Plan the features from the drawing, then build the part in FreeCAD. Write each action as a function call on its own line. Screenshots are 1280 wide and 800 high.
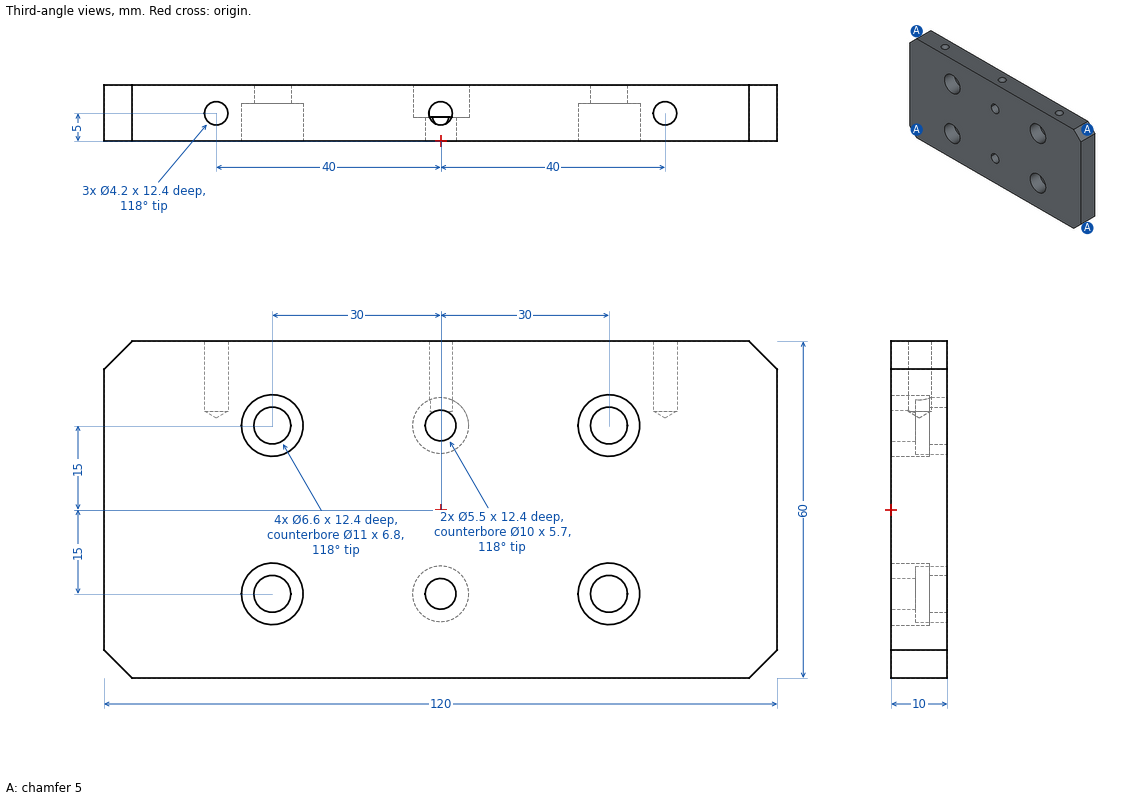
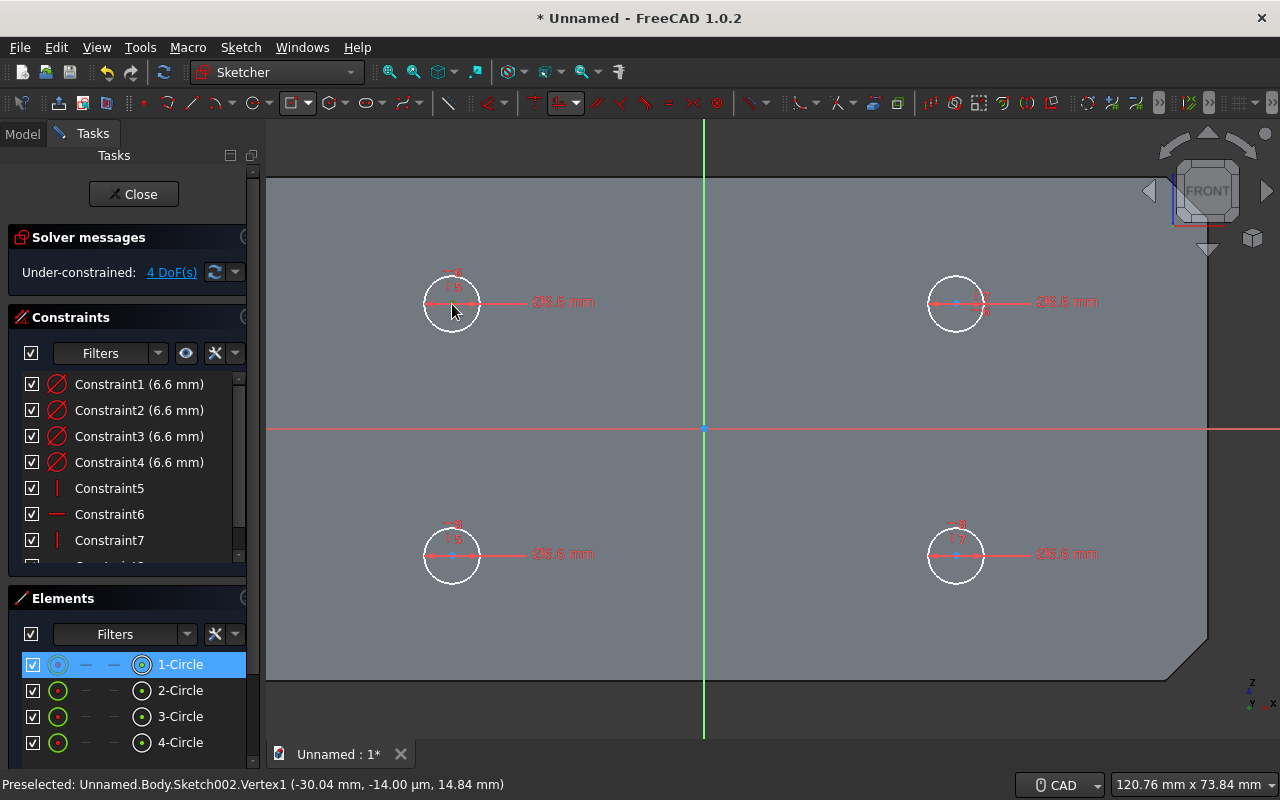
key(l)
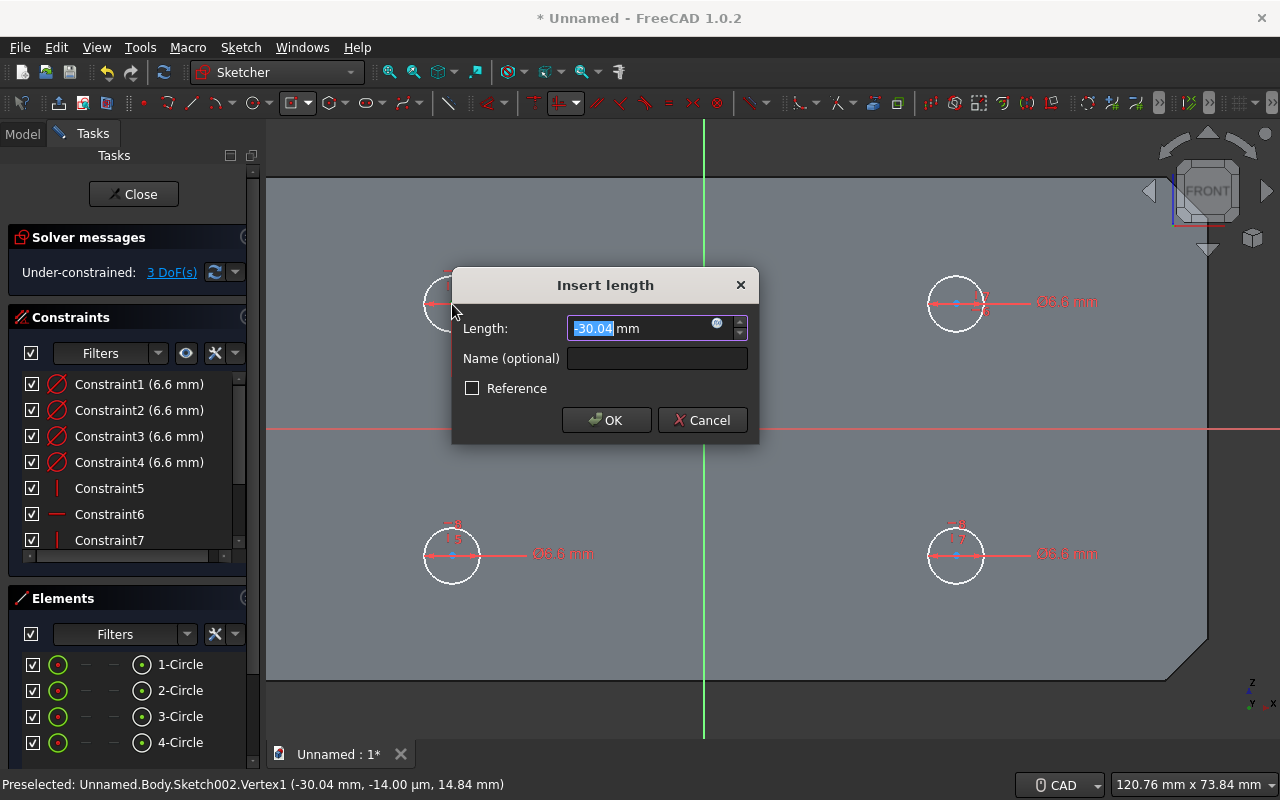
text(-30)
key(Return)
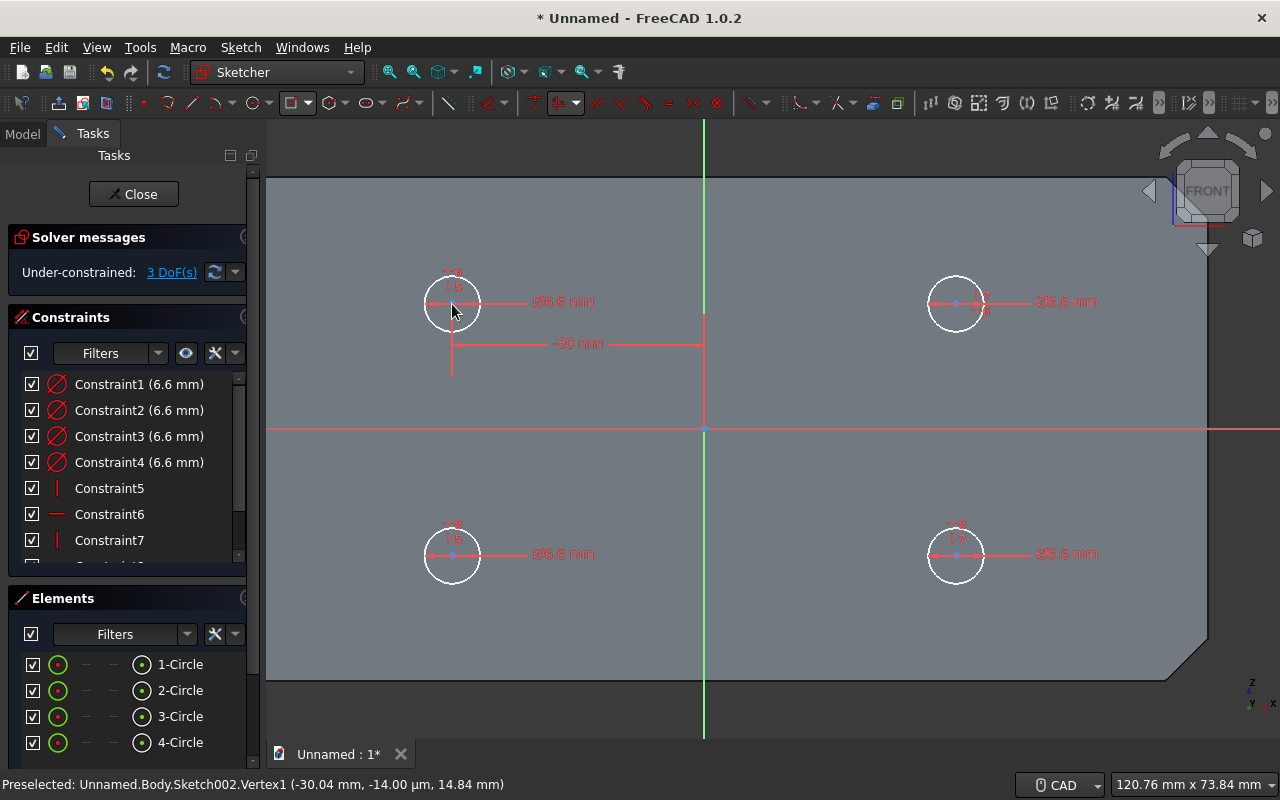
click(452, 304)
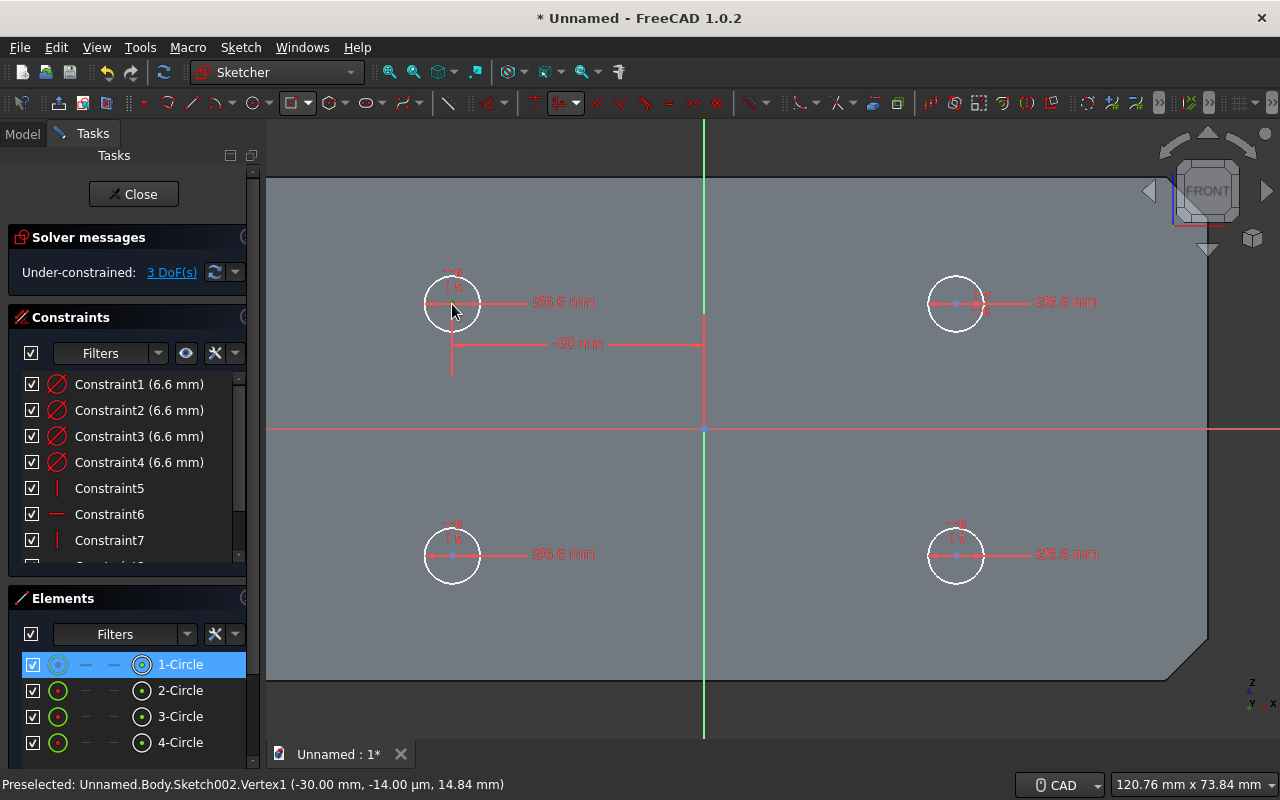
key(i)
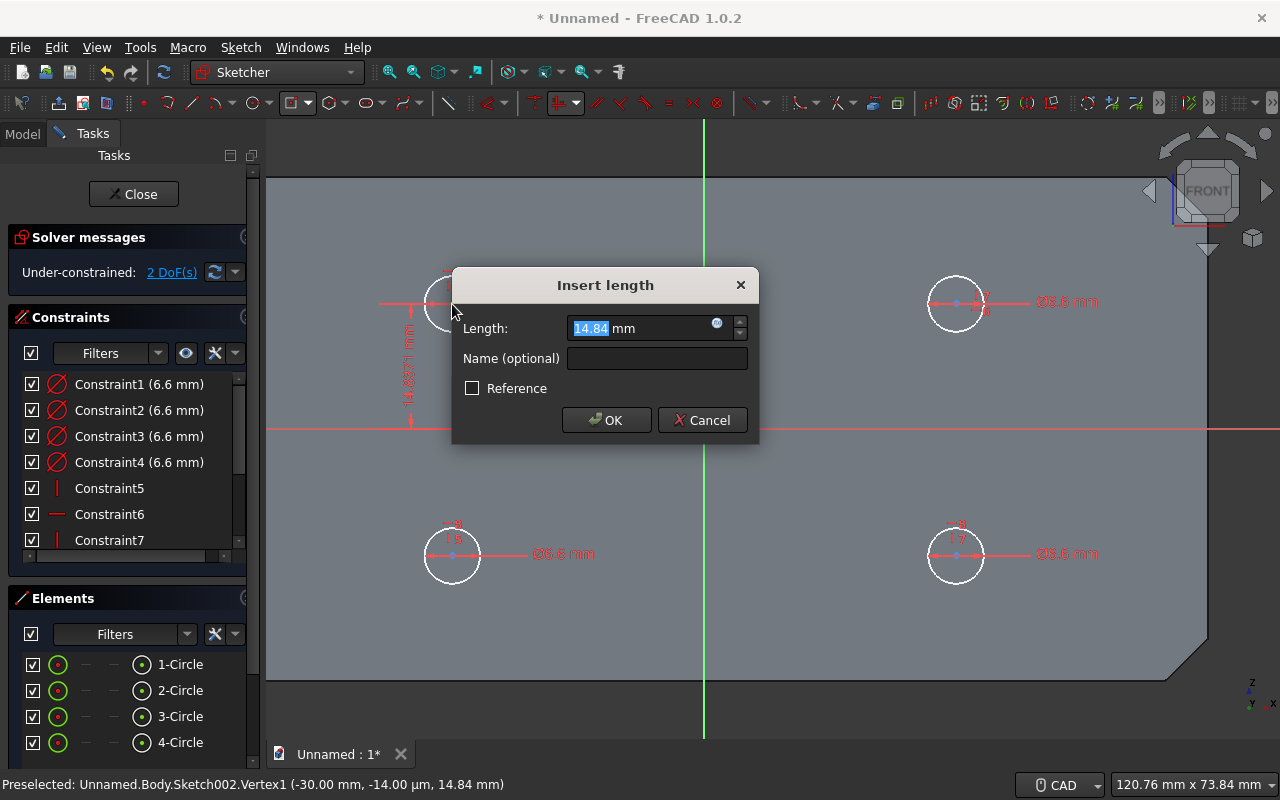
text(15)
key(Return)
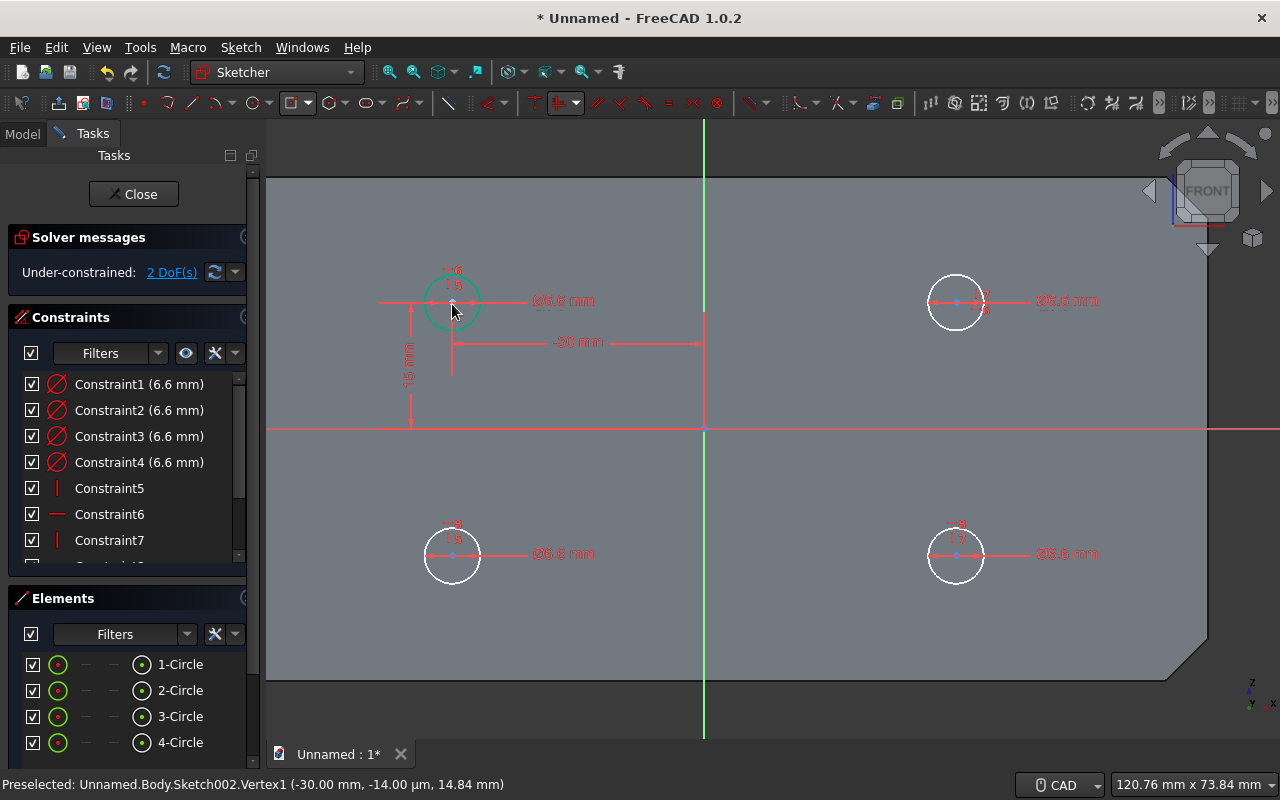
click(452, 556)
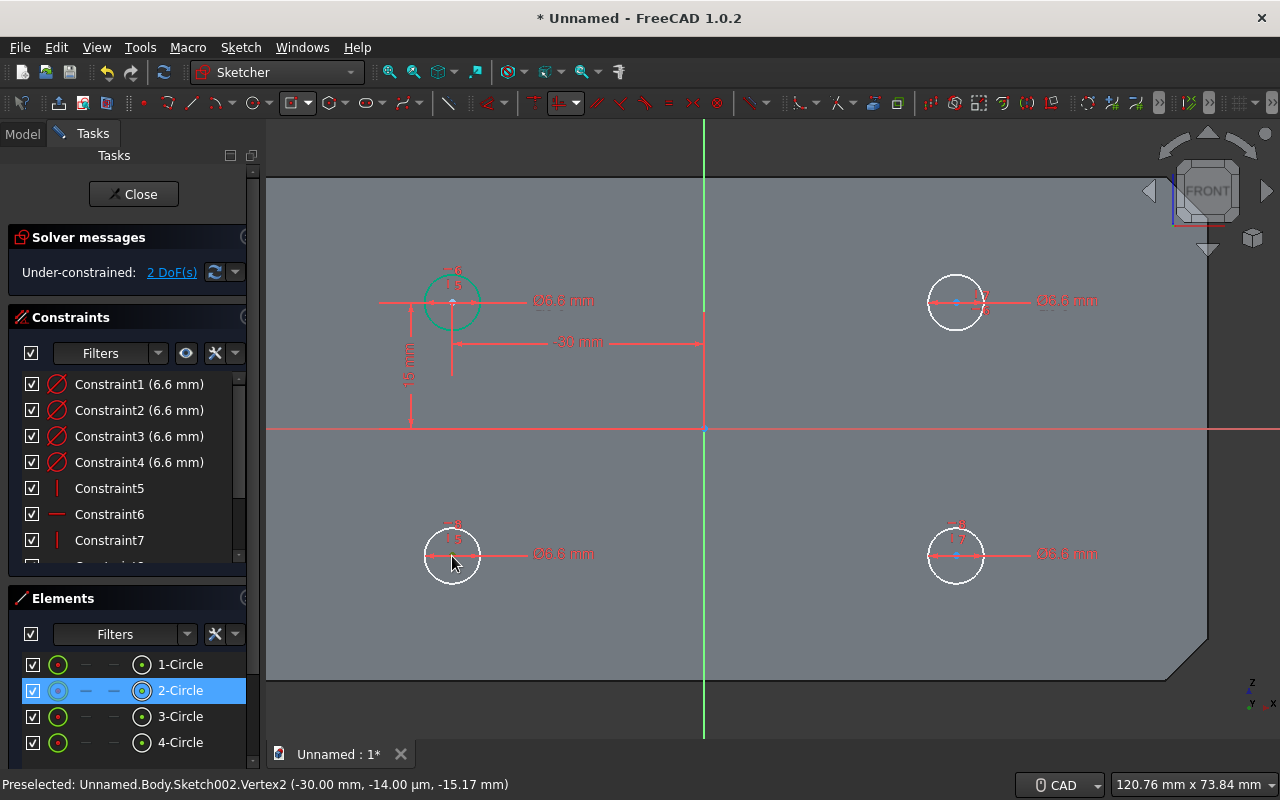
click(506, 104)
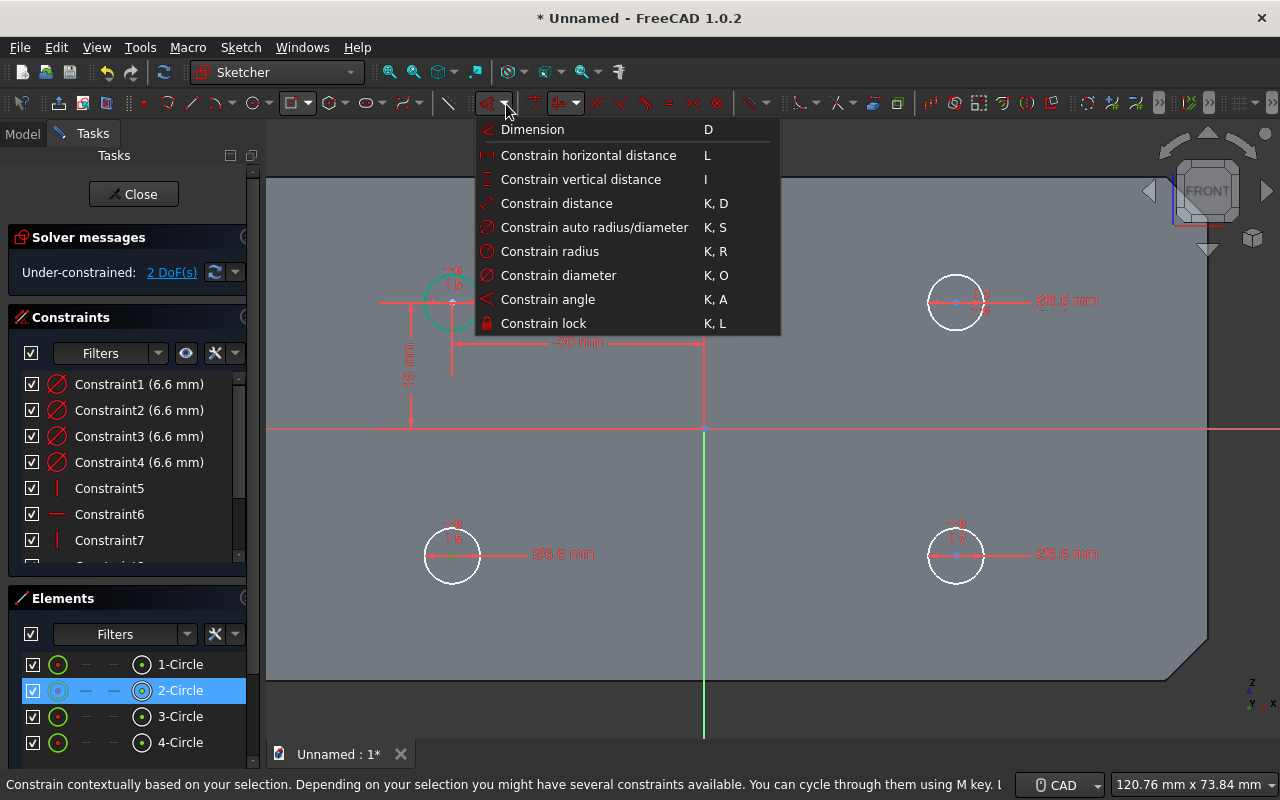
click(628, 179)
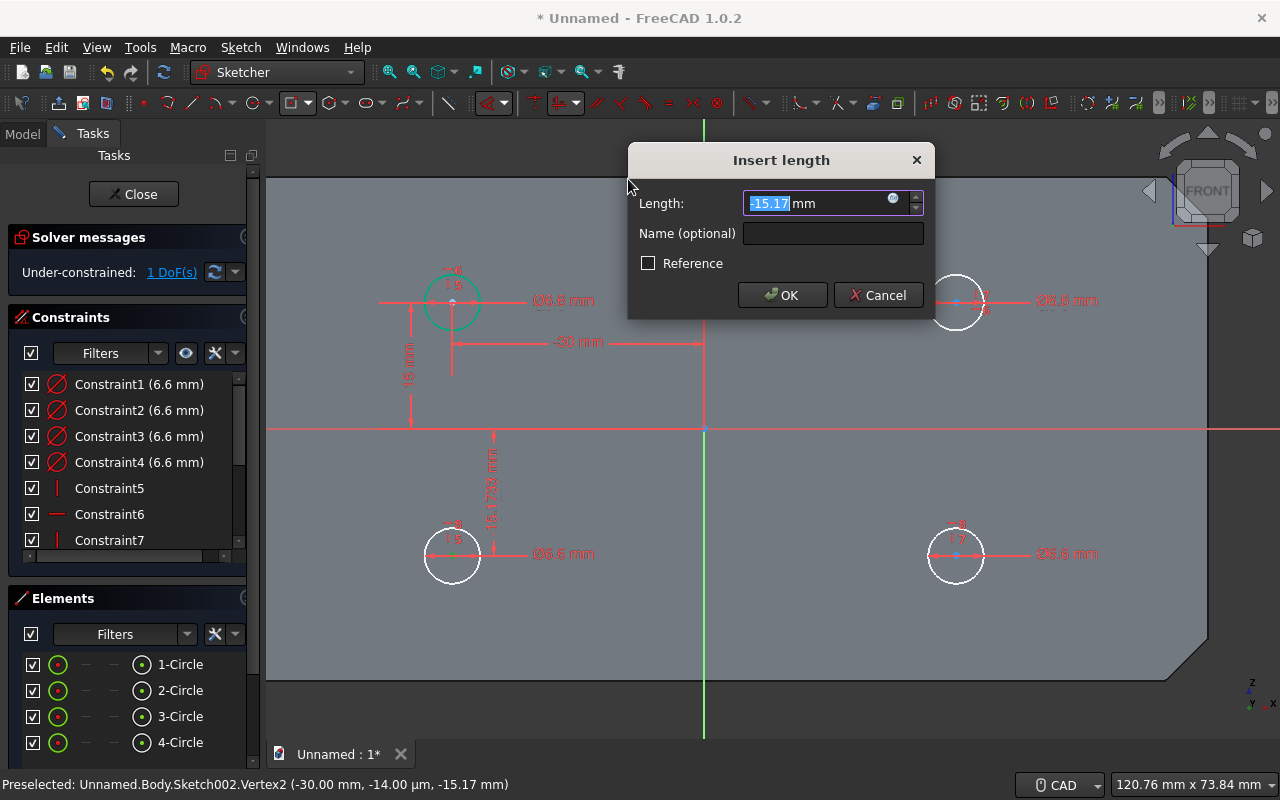
text(-15)
key(Return)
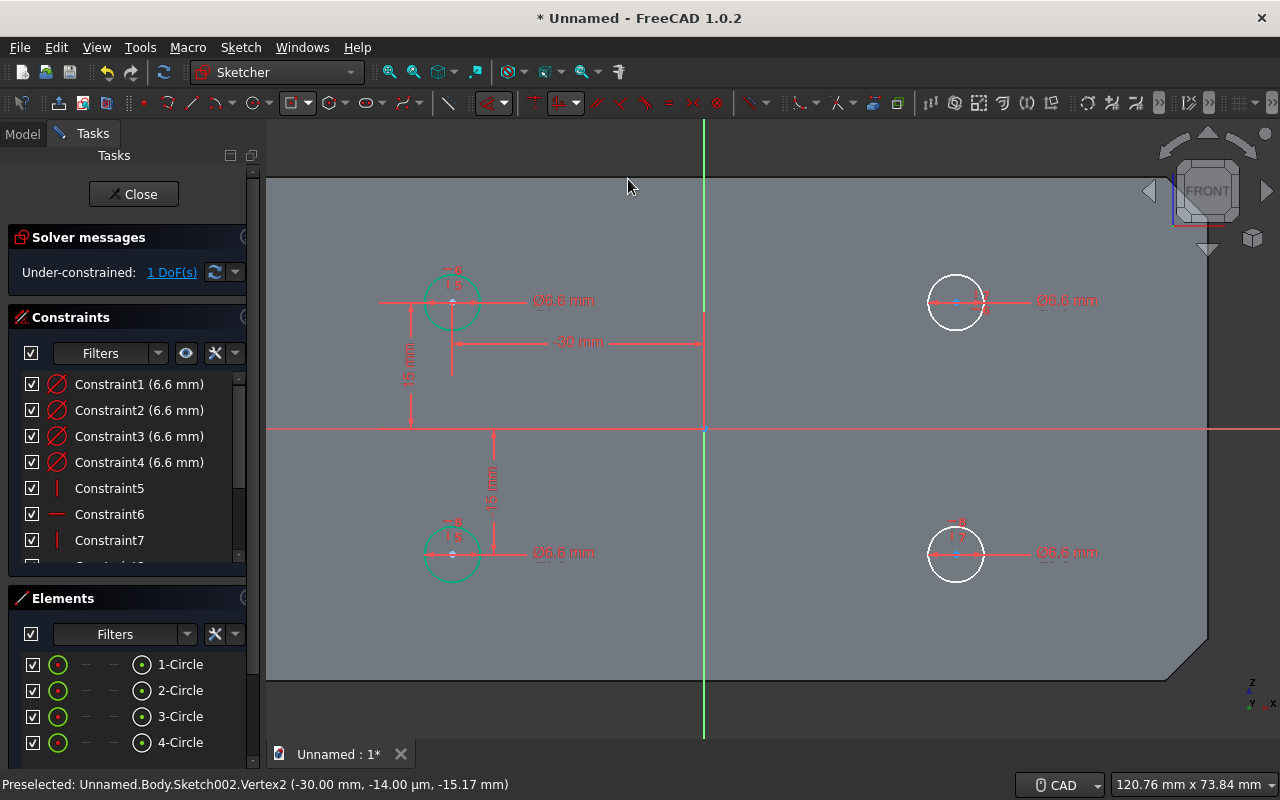
click(956, 303)